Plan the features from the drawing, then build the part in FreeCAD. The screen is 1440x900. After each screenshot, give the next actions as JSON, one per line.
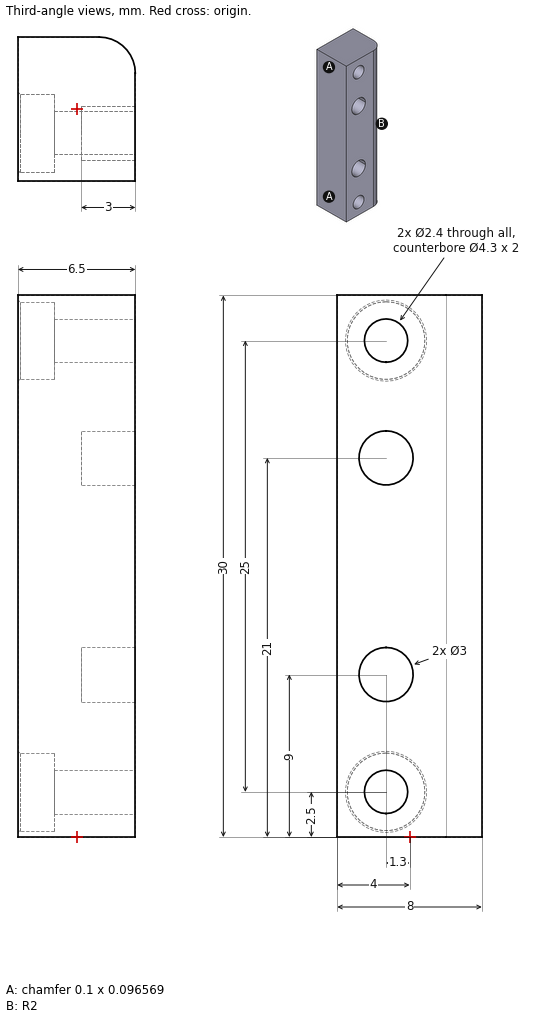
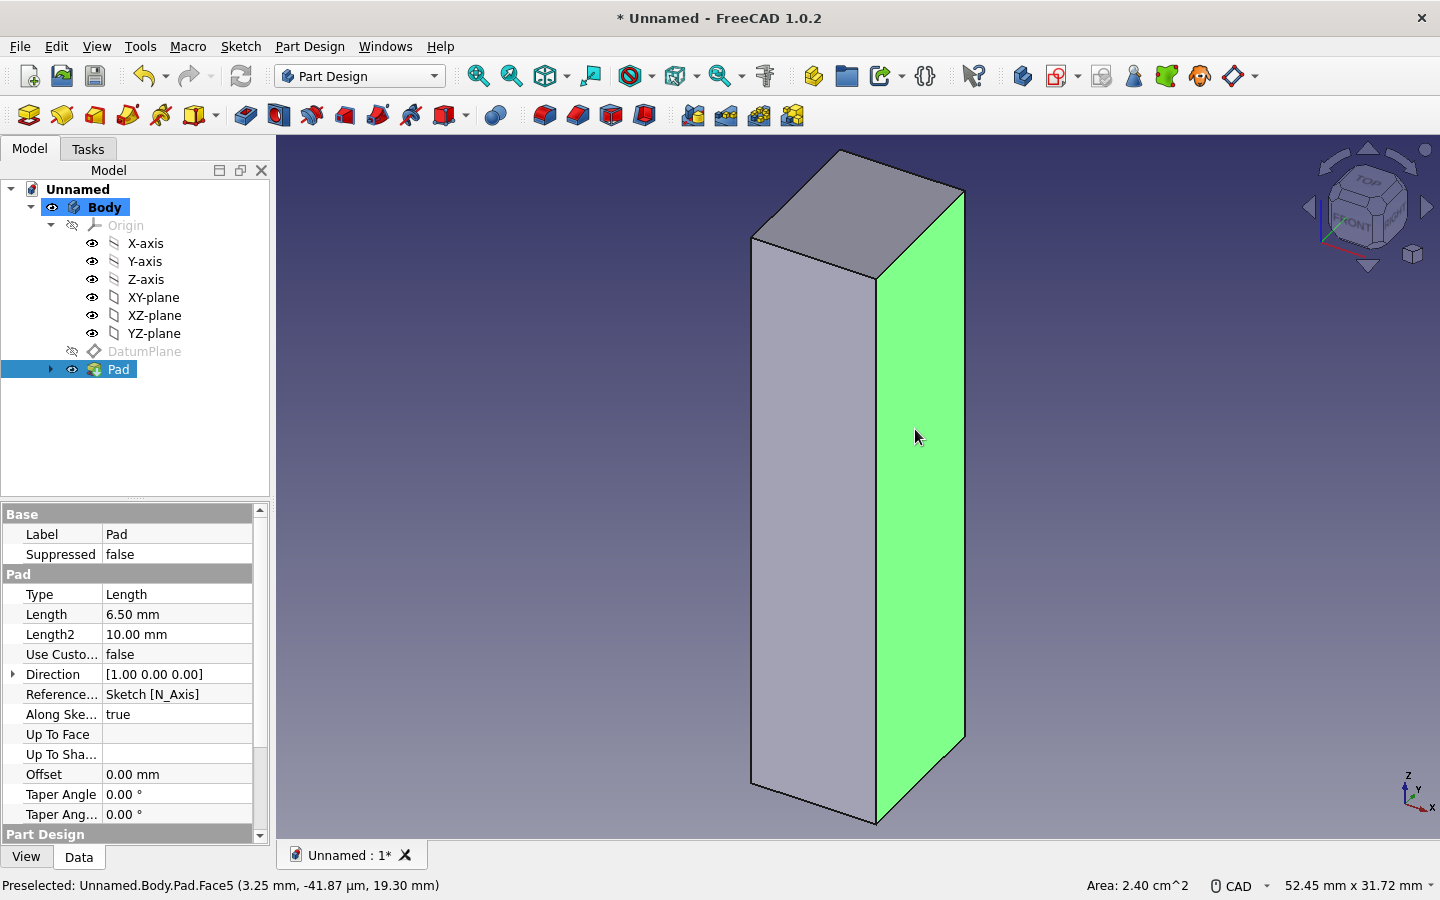
{"action": "left_click", "coordinate": [1056, 76]}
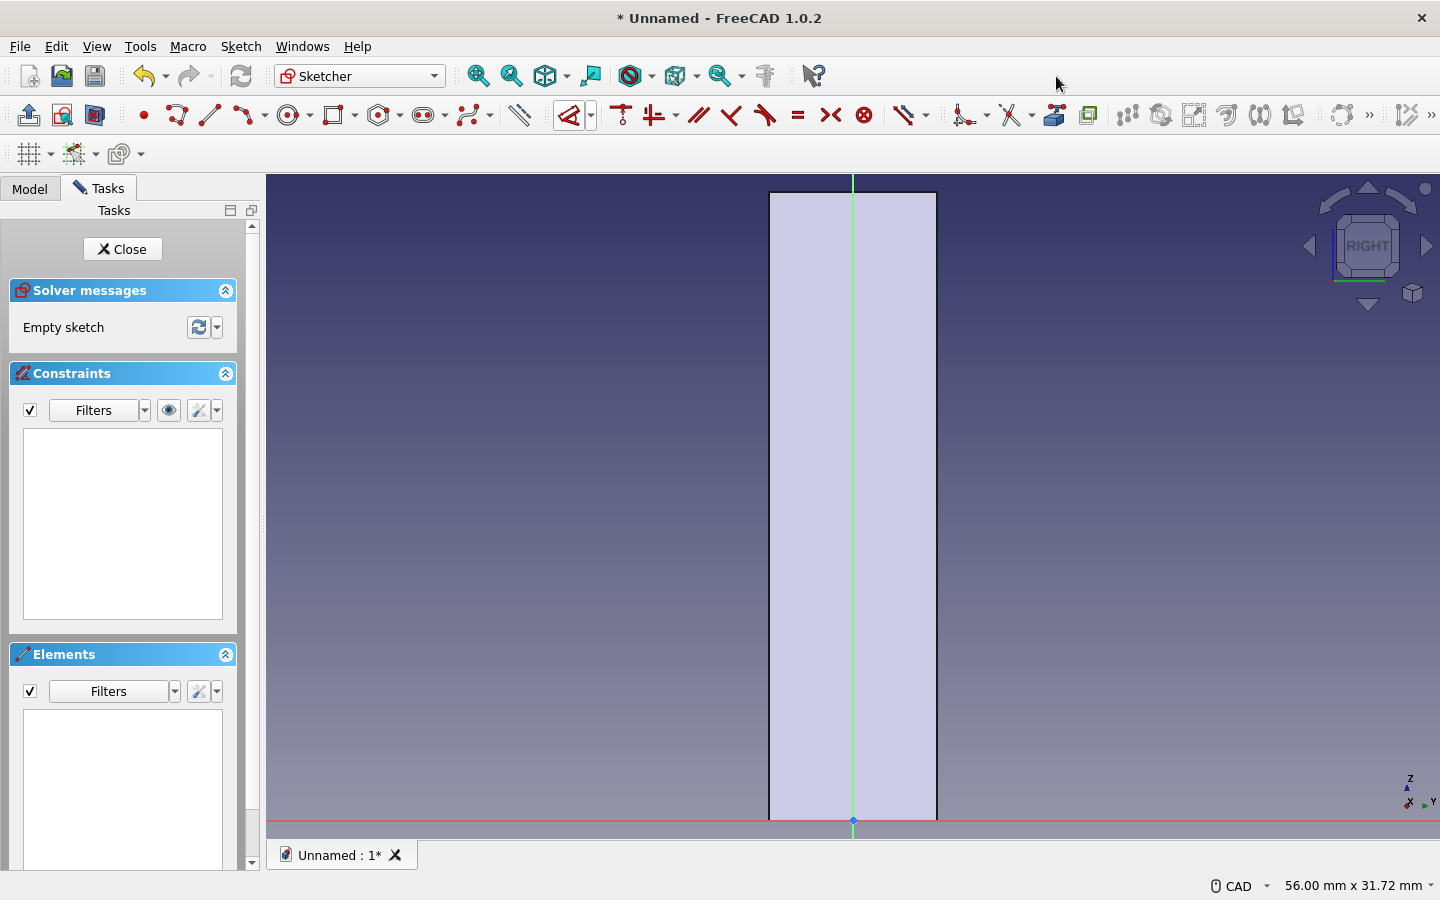
{"action": "scroll", "coordinate": [598, 202], "scroll_direction": "down", "scroll_amount": 1}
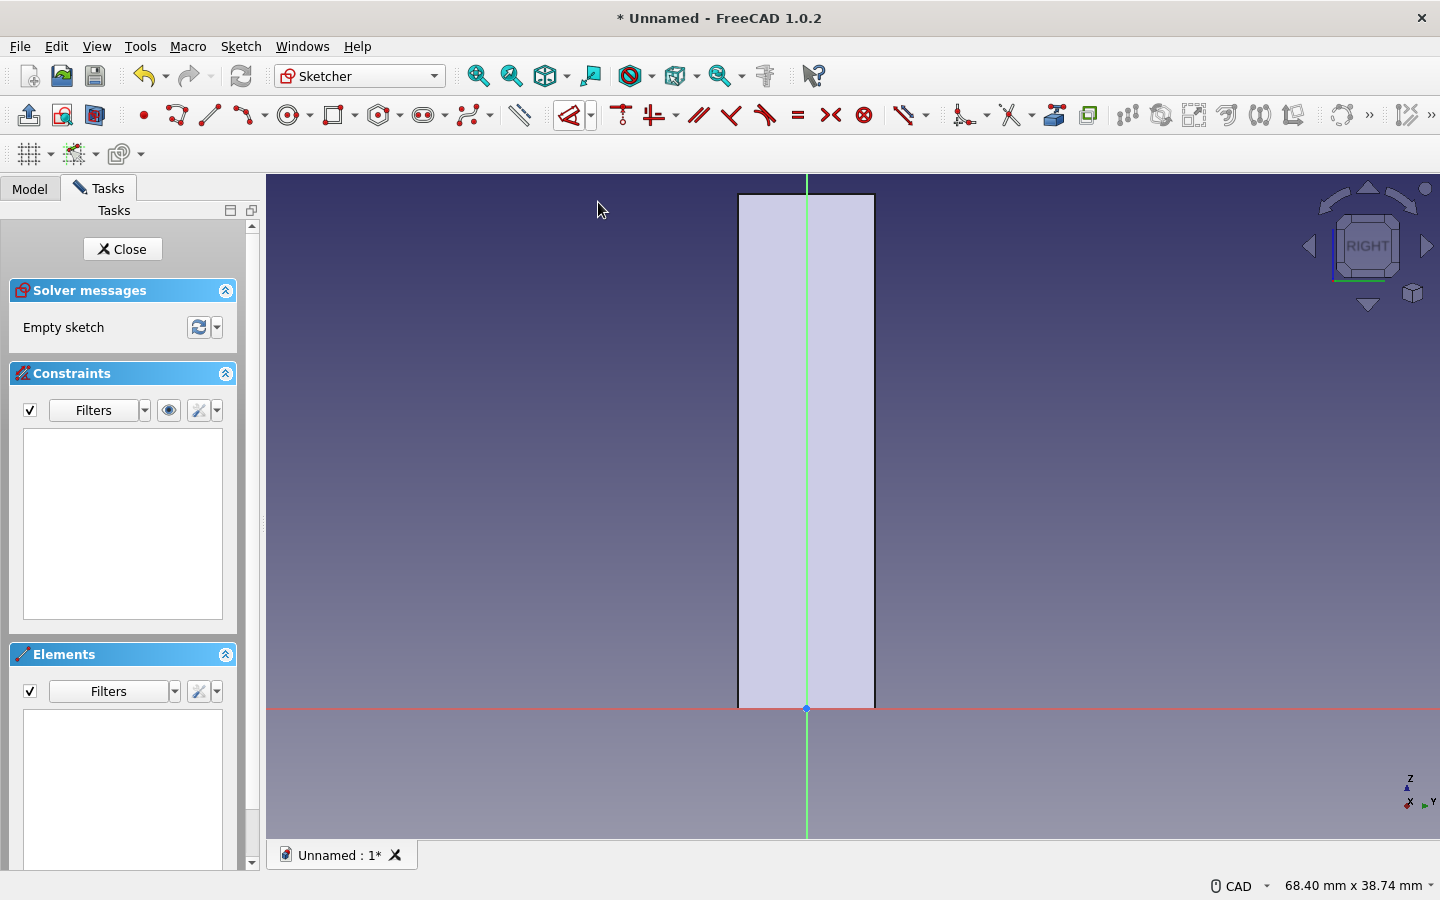
{"action": "left_click", "coordinate": [288, 116]}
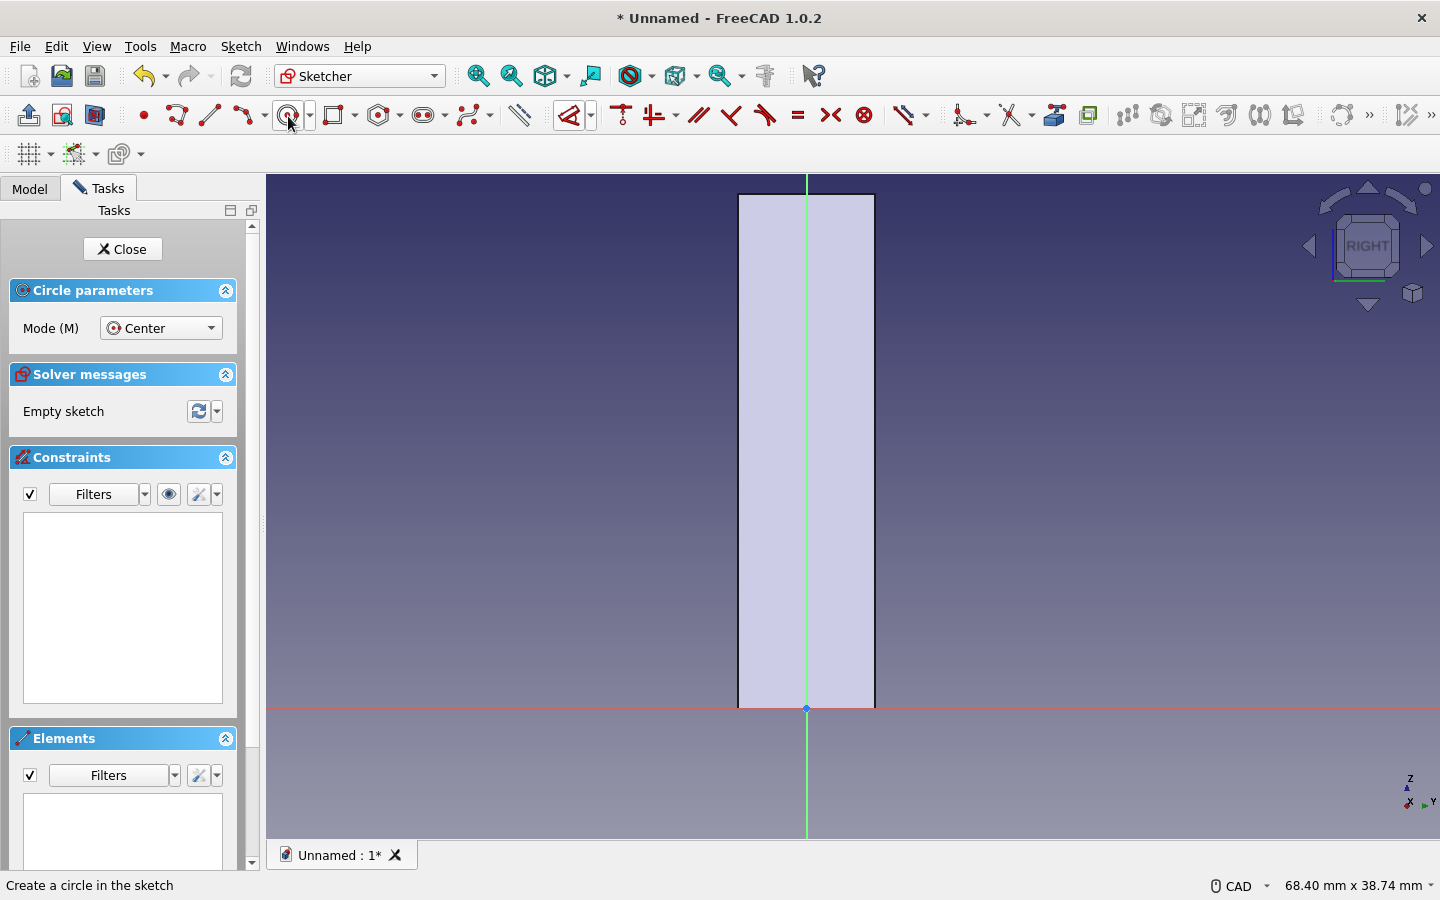
{"action": "left_click", "coordinate": [785, 554]}
{"action": "mouse_move", "coordinate": [766, 536]}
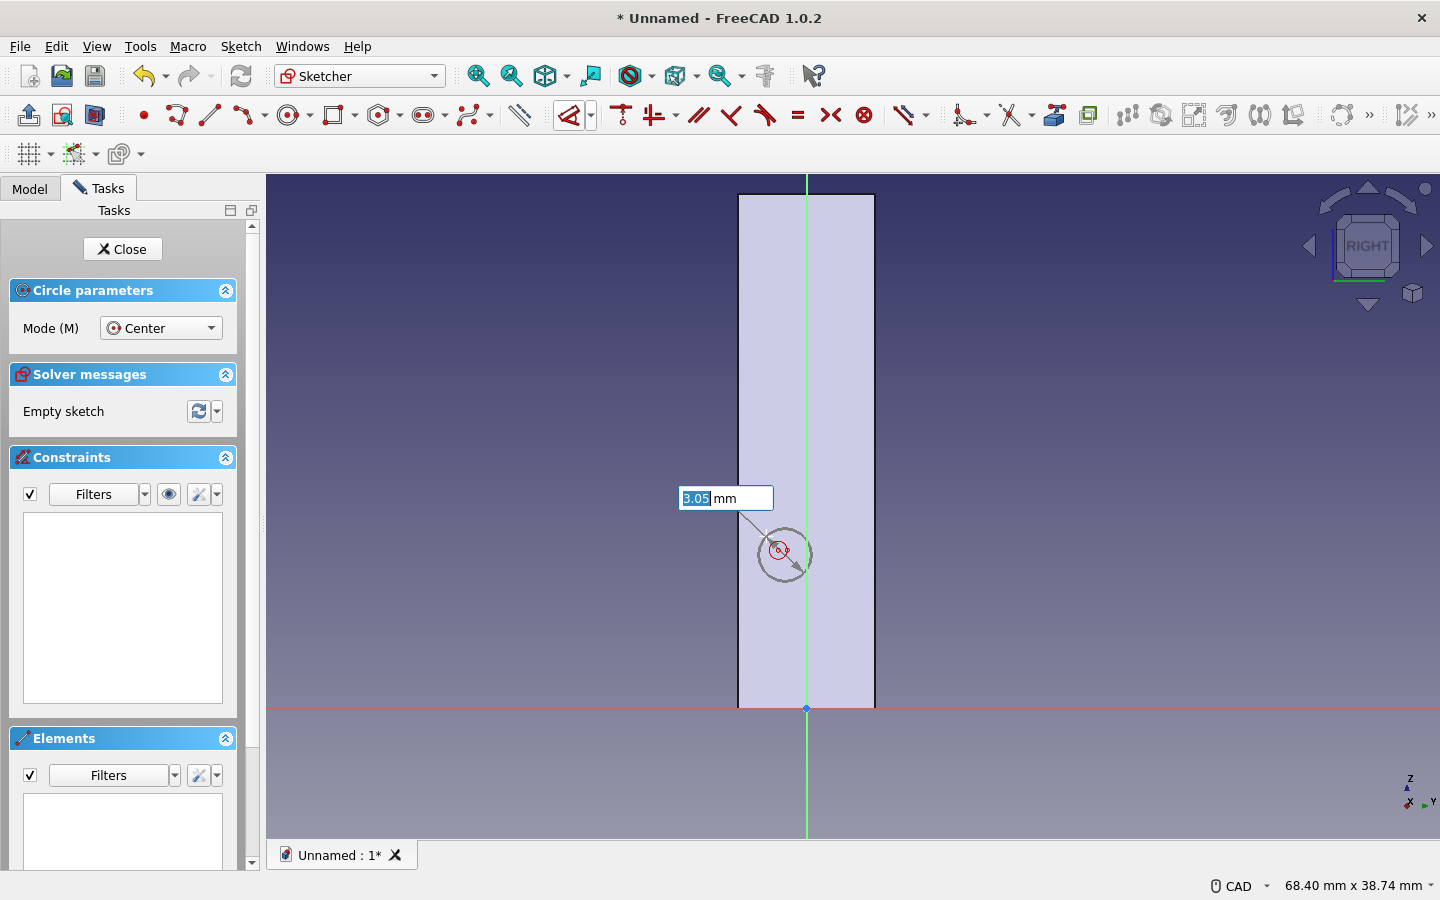
{"action": "type", "text": "3"}
{"action": "key", "text": "Return"}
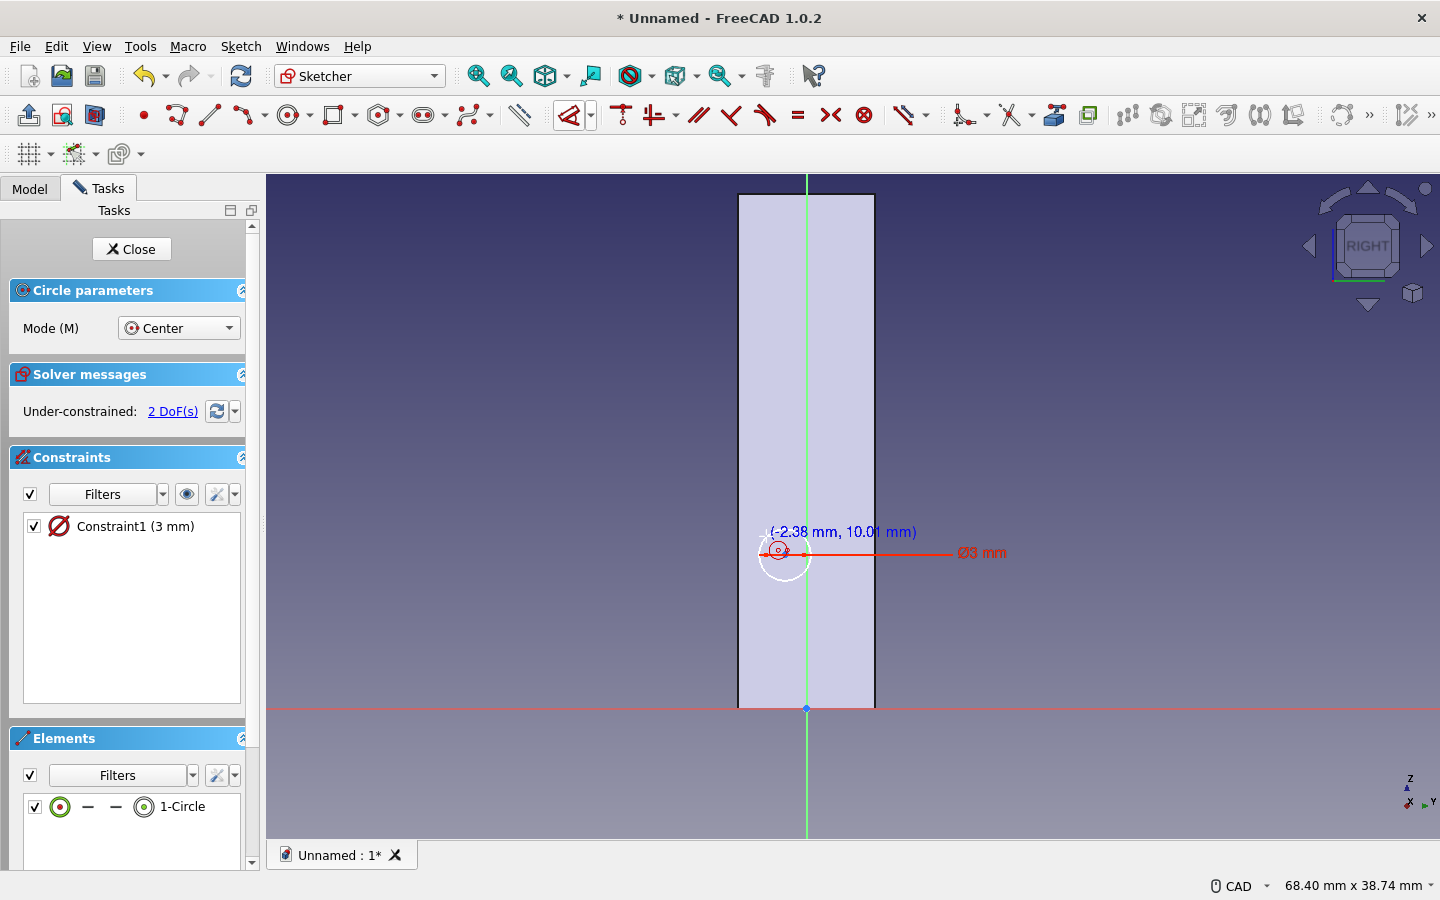
{"action": "left_click", "coordinate": [785, 348]}
{"action": "mouse_move", "coordinate": [766, 330]}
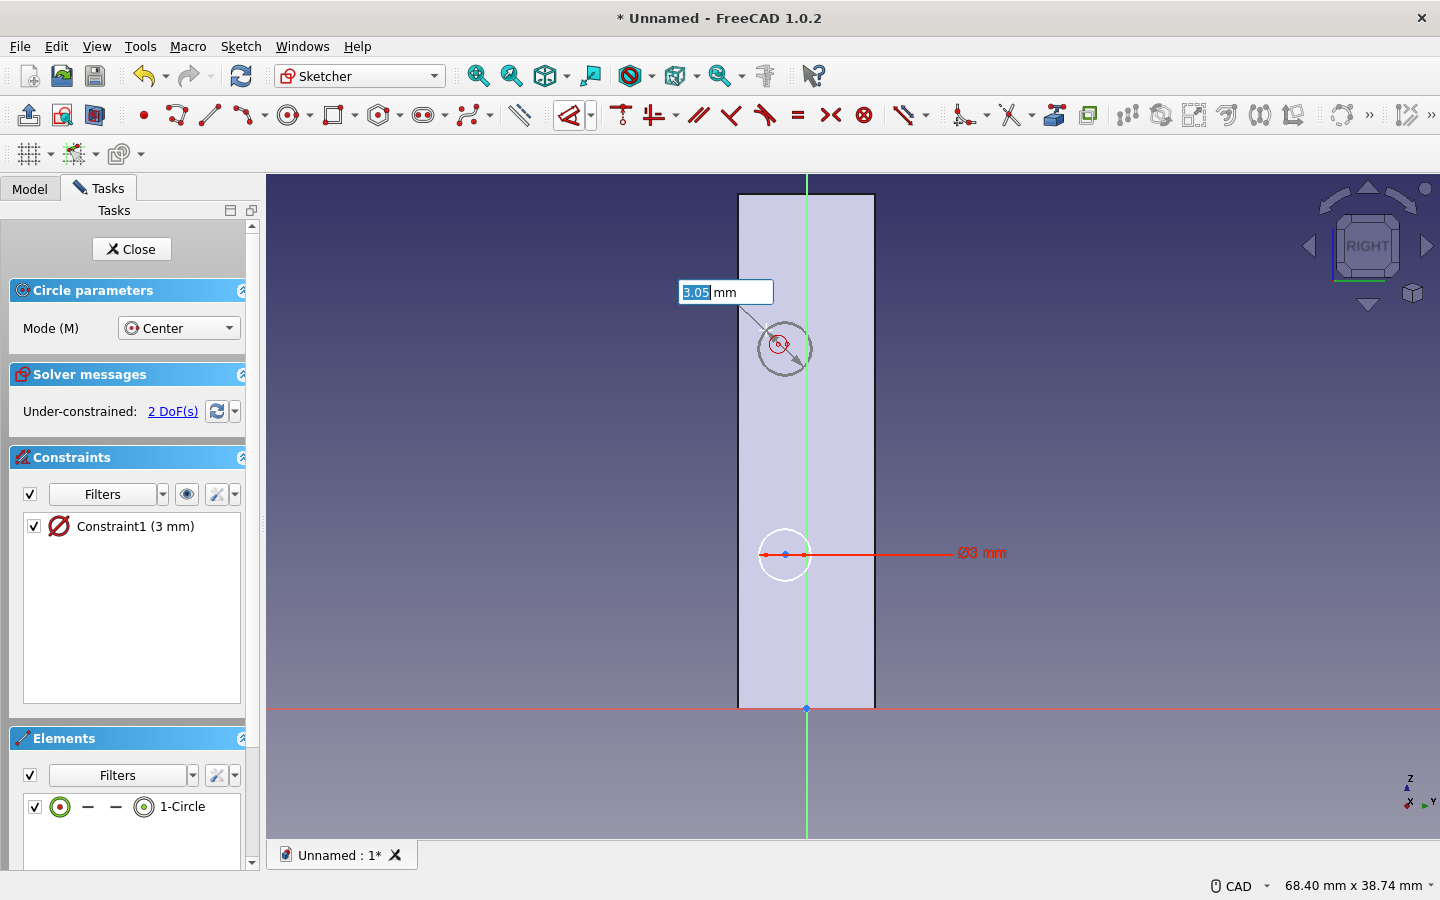
{"action": "type", "text": "3"}
{"action": "key", "text": "Return"}
{"action": "key", "text": "Escape"}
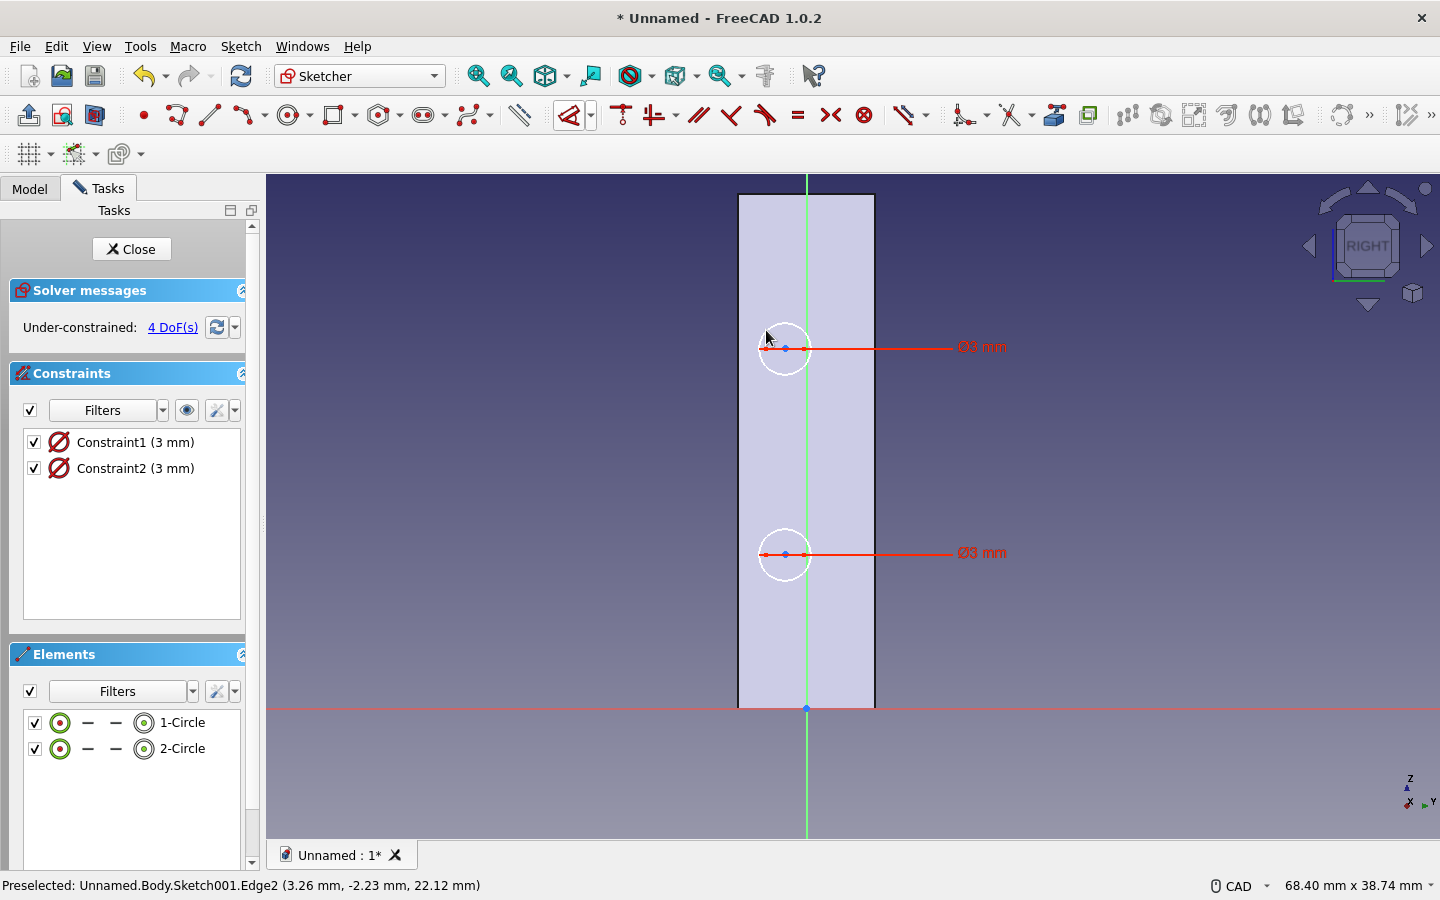
{"action": "left_click", "coordinate": [785, 555]}